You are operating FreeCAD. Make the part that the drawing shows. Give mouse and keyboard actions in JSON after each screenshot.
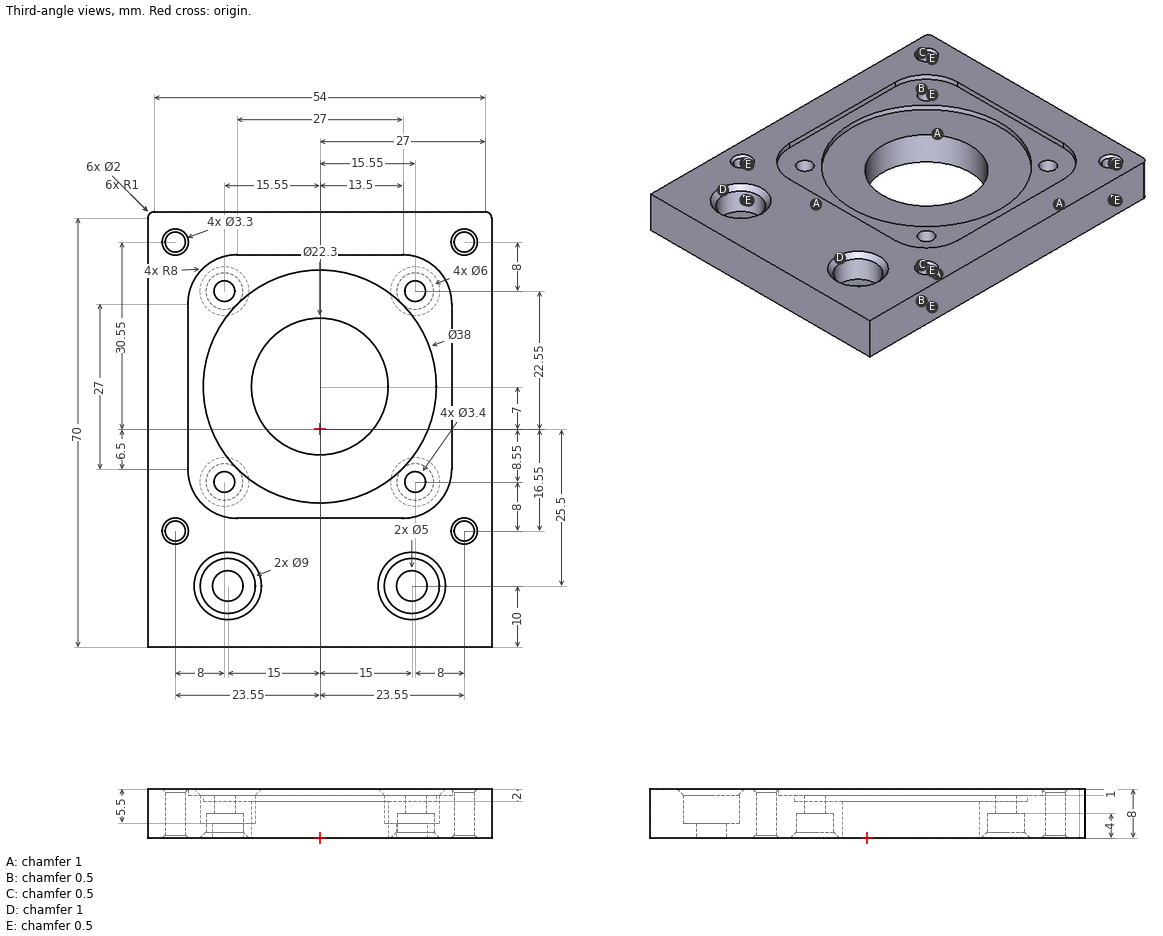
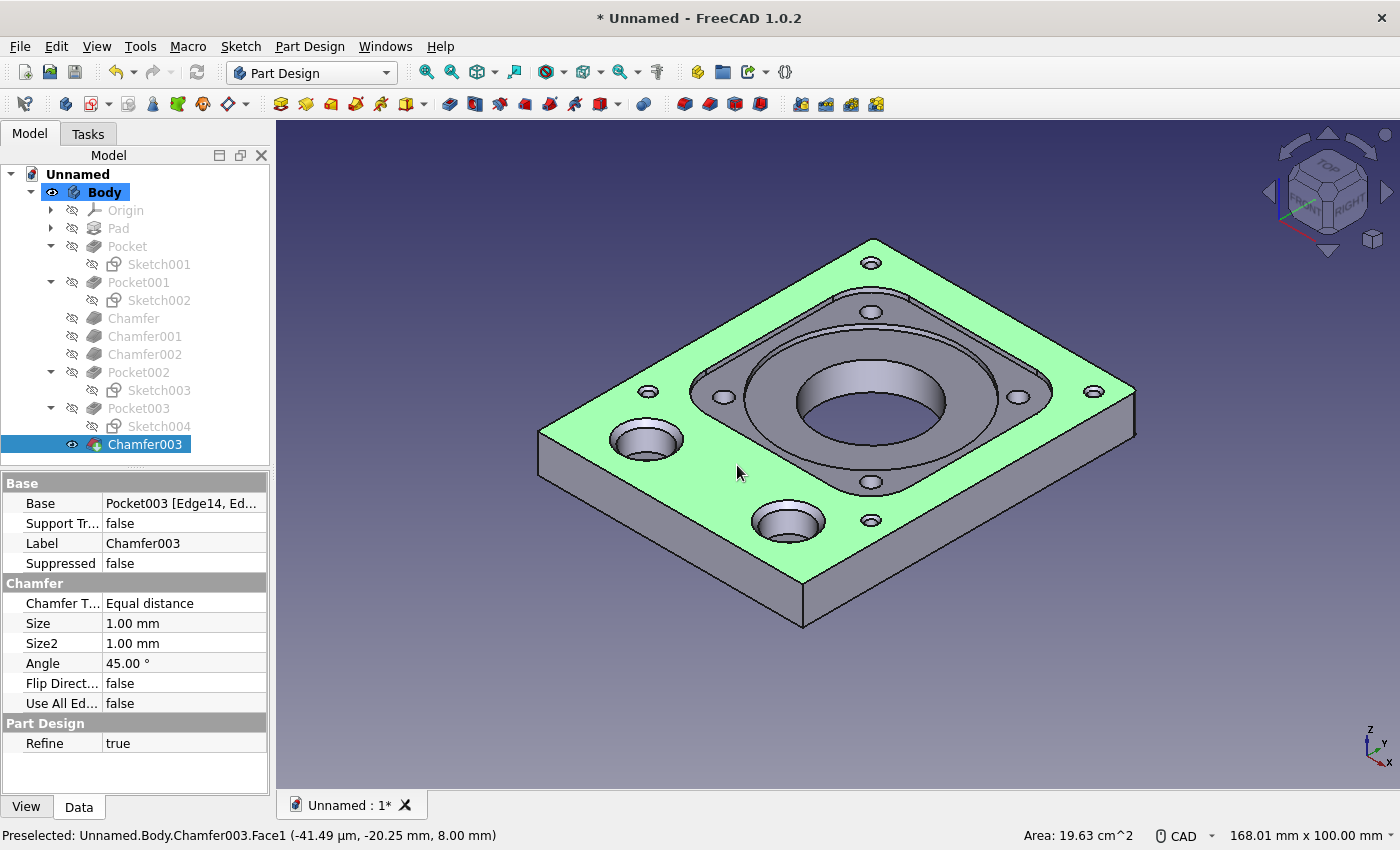
{"action": "left_click", "coordinate": [90, 104]}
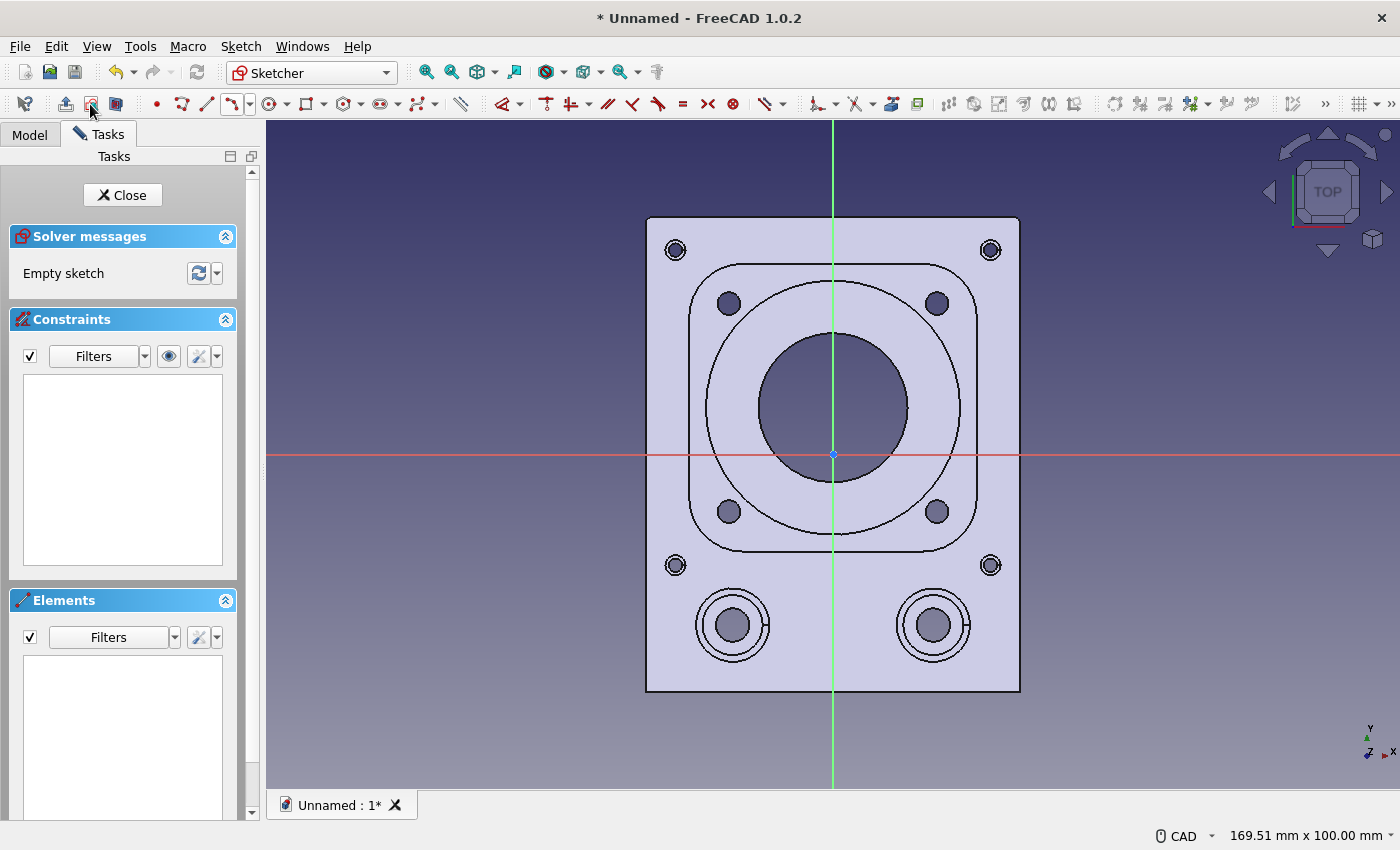
{"action": "key", "text": "g c"}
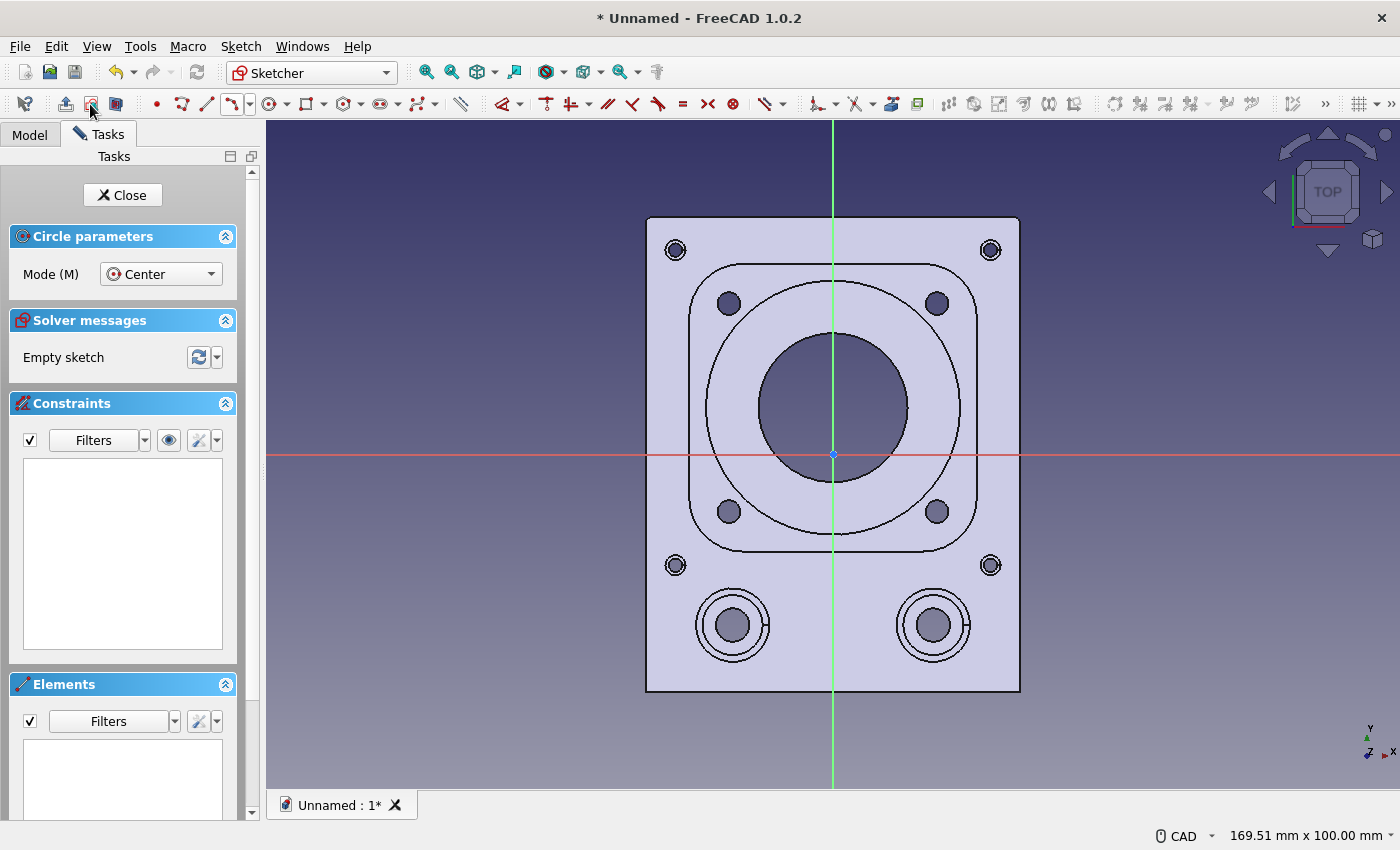
{"action": "scroll", "coordinate": [675, 250], "scroll_direction": "up", "scroll_amount": 4}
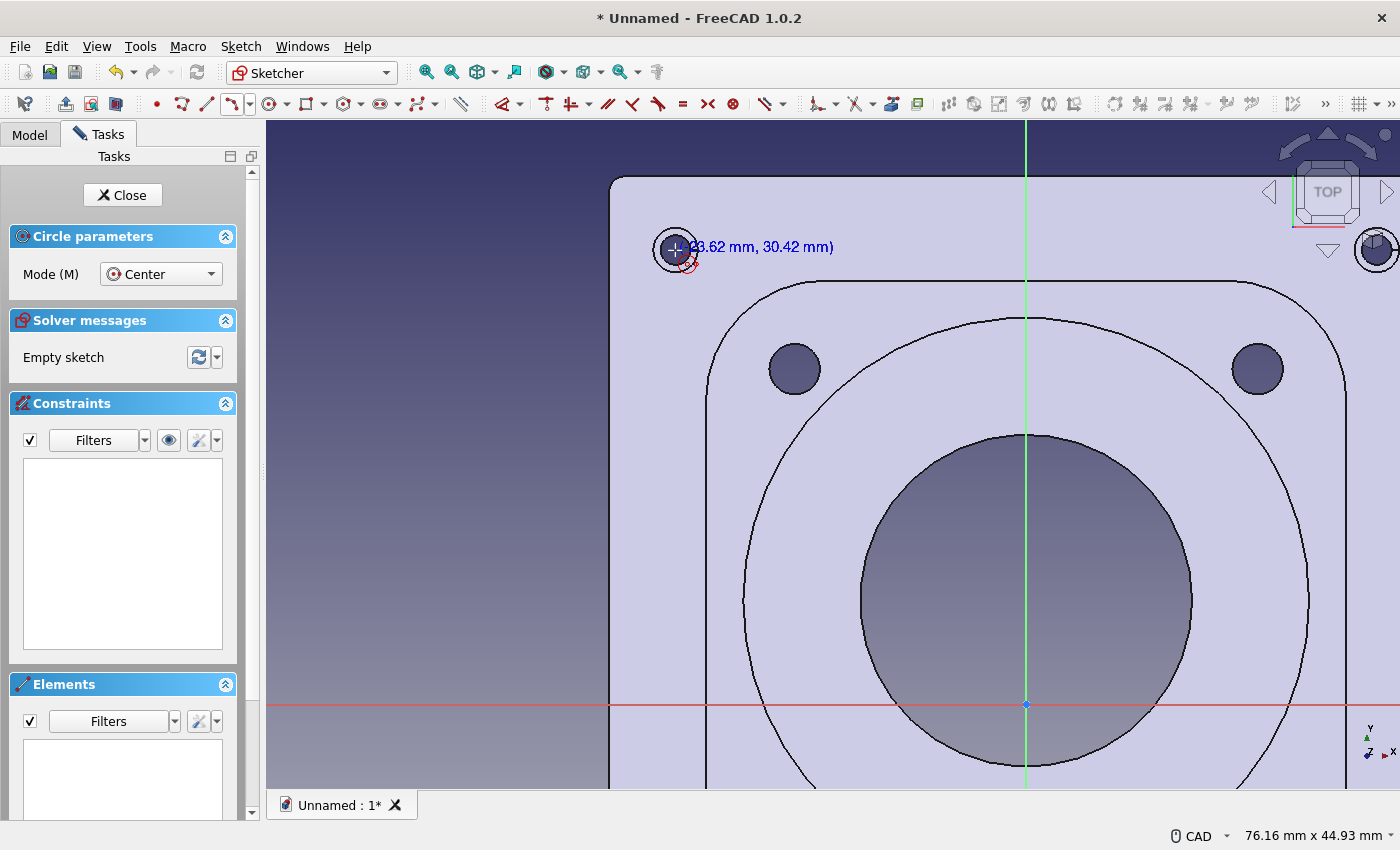
{"action": "left_click", "coordinate": [676, 250]}
{"action": "left_click", "coordinate": [693, 233]}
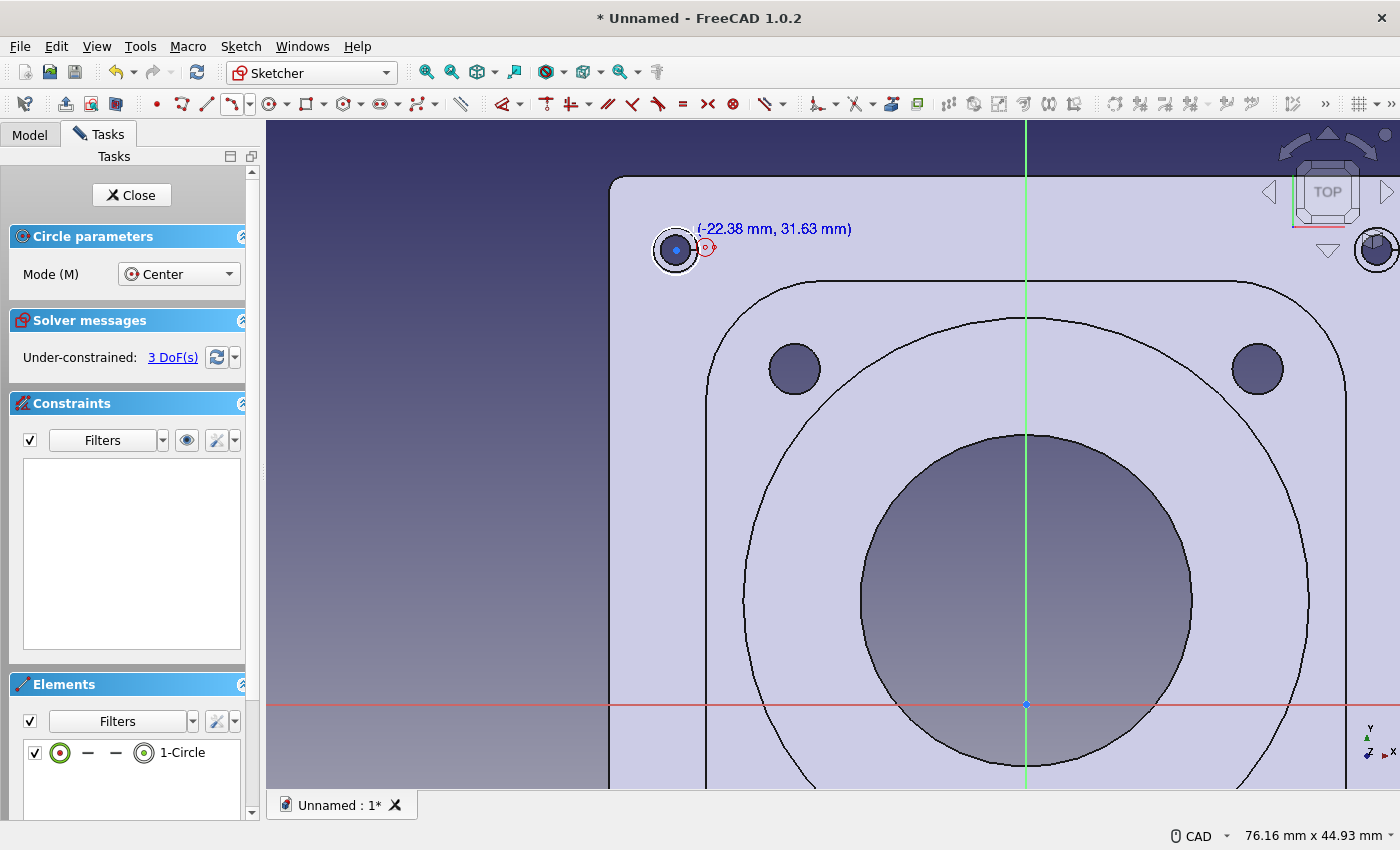
{"action": "scroll", "coordinate": [446, 277], "scroll_direction": "down", "scroll_amount": 3}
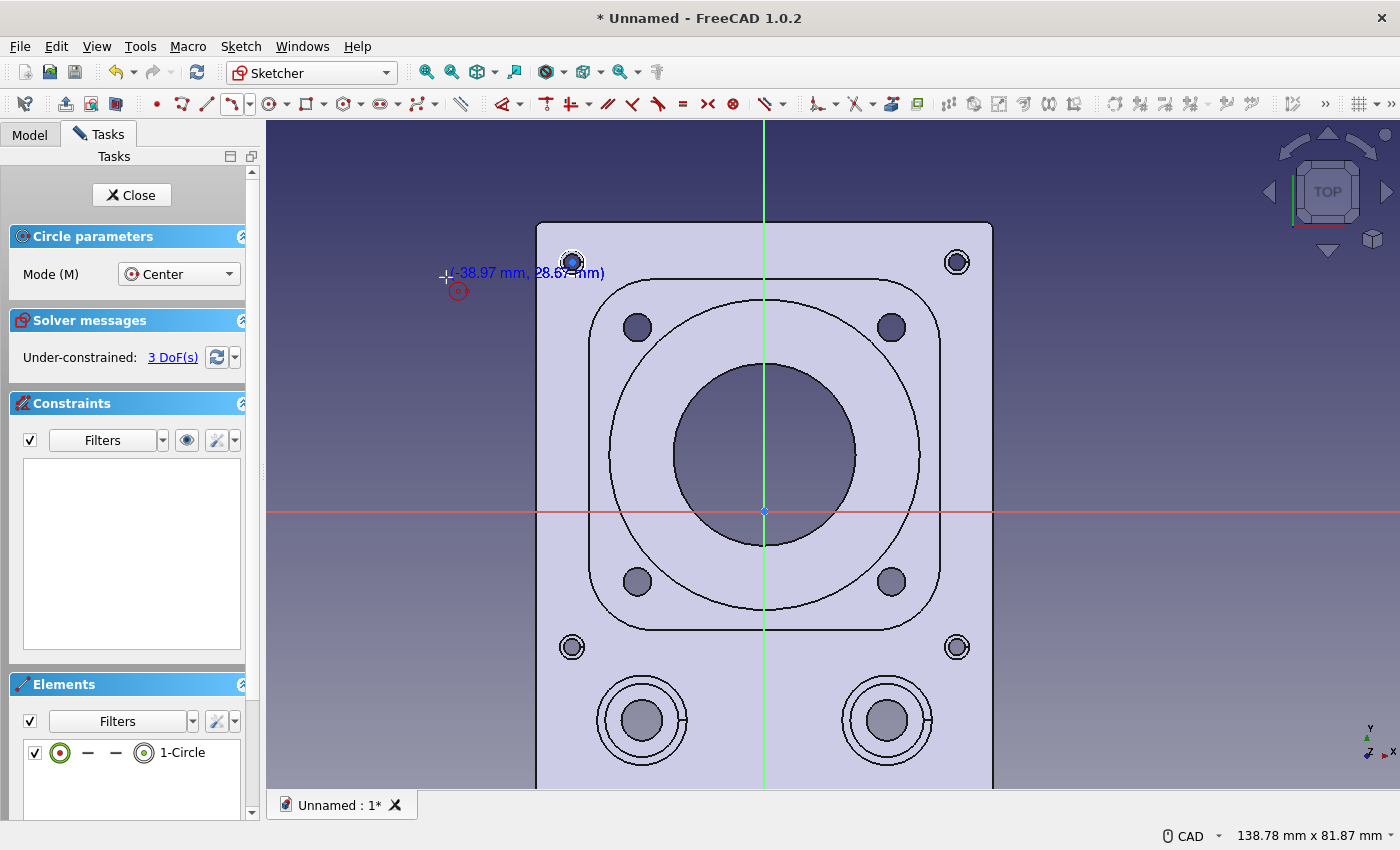
{"action": "scroll", "coordinate": [957, 262], "scroll_direction": "up", "scroll_amount": 3}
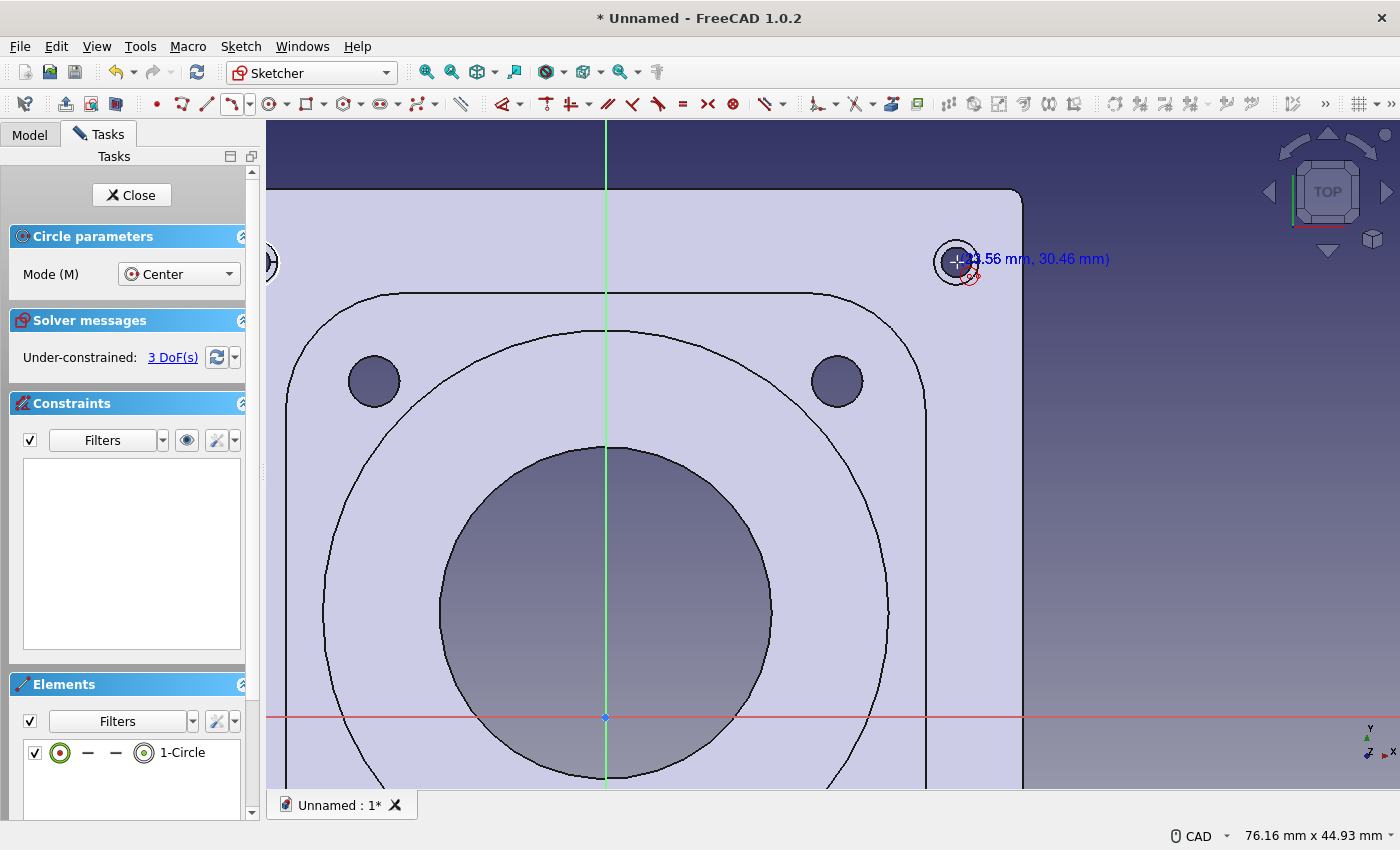
{"action": "left_click", "coordinate": [956, 262]}
{"action": "left_click", "coordinate": [974, 245]}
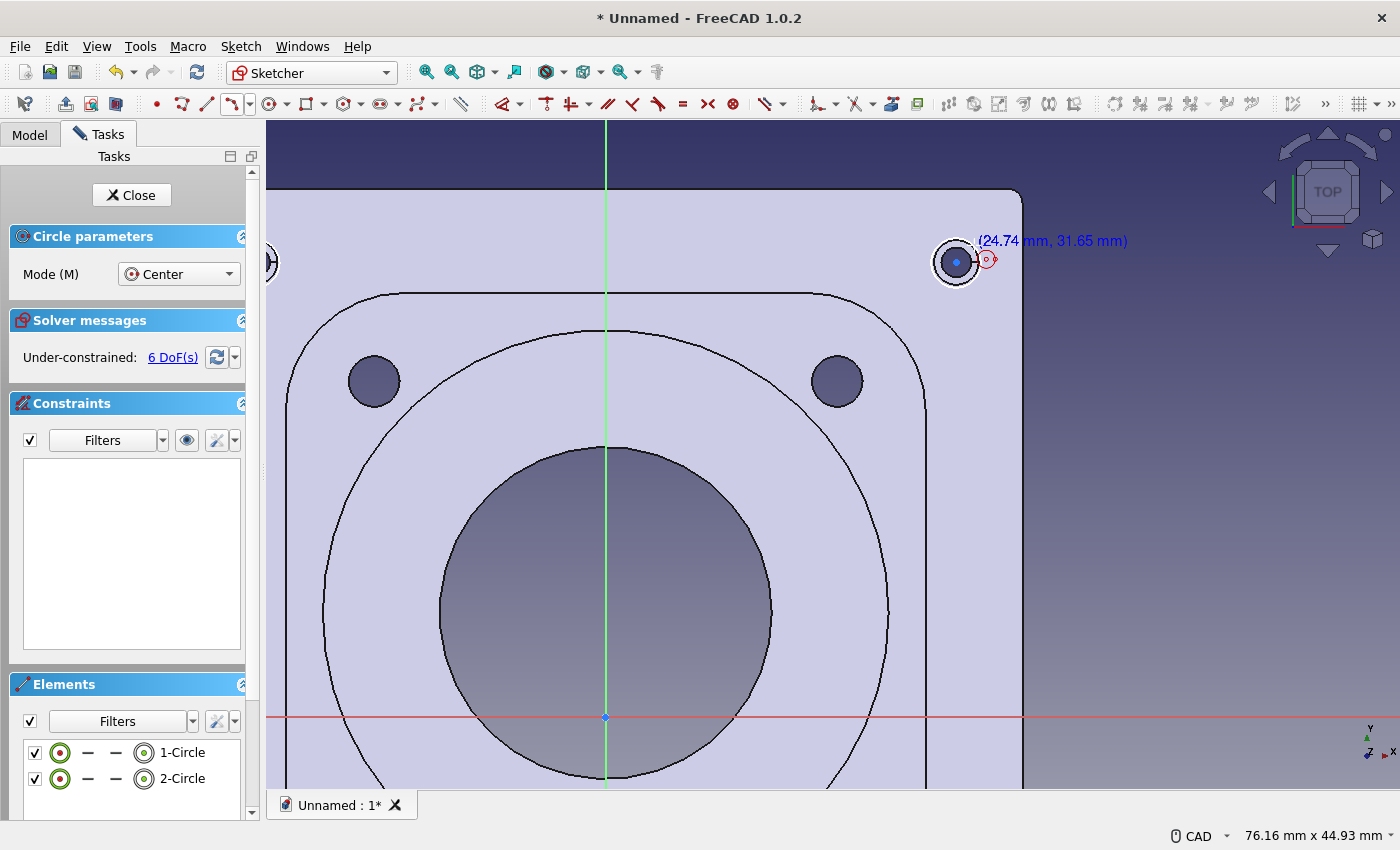
{"action": "scroll", "coordinate": [958, 262], "scroll_direction": "down", "scroll_amount": 3}